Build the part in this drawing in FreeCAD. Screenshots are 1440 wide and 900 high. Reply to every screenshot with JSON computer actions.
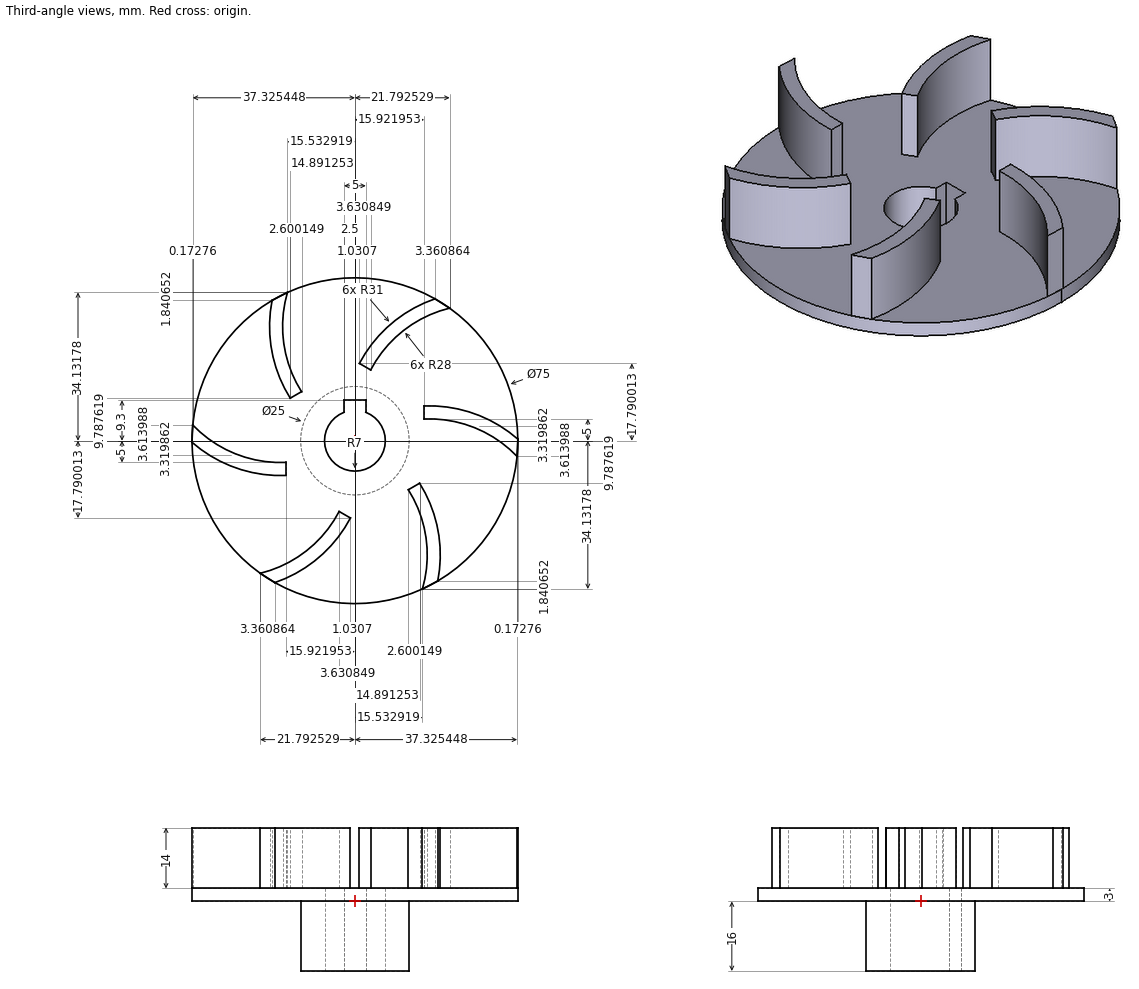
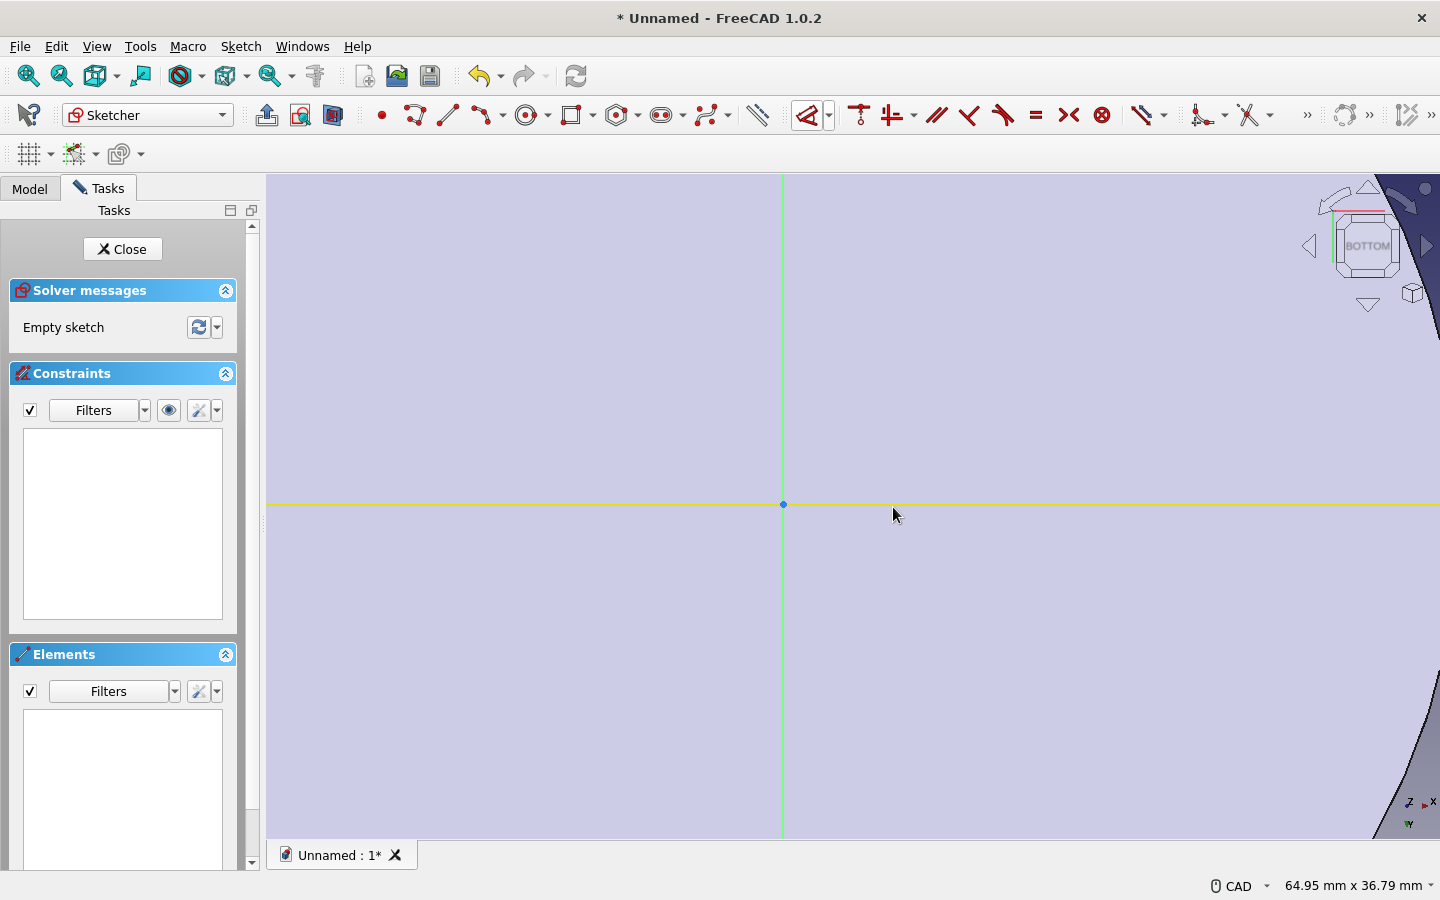
{"action": "key", "text": "g c"}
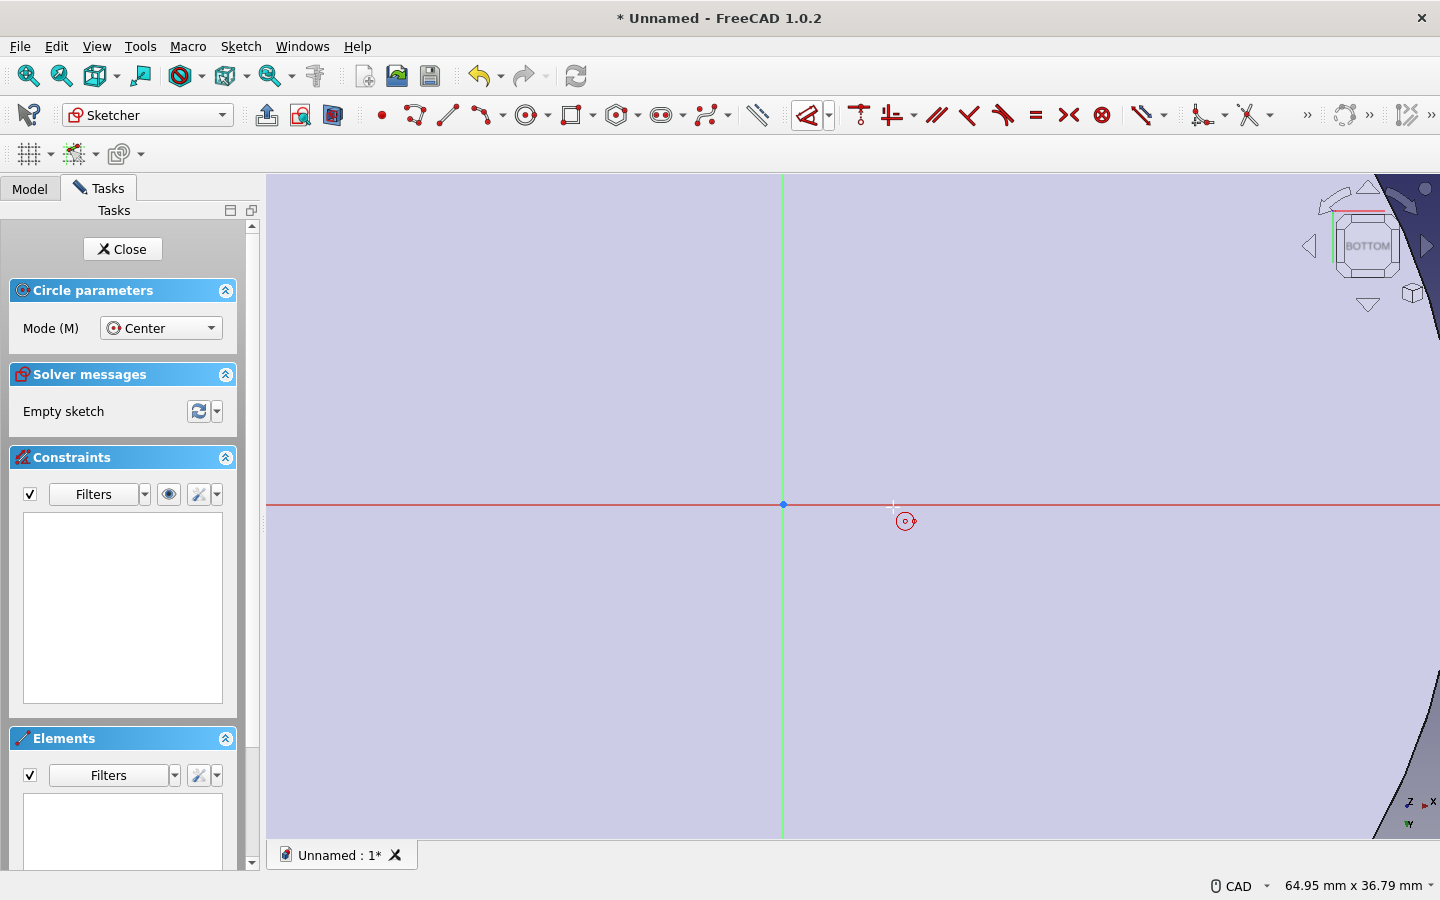
{"action": "left_click", "coordinate": [783, 505]}
{"action": "mouse_move", "coordinate": [943, 345]}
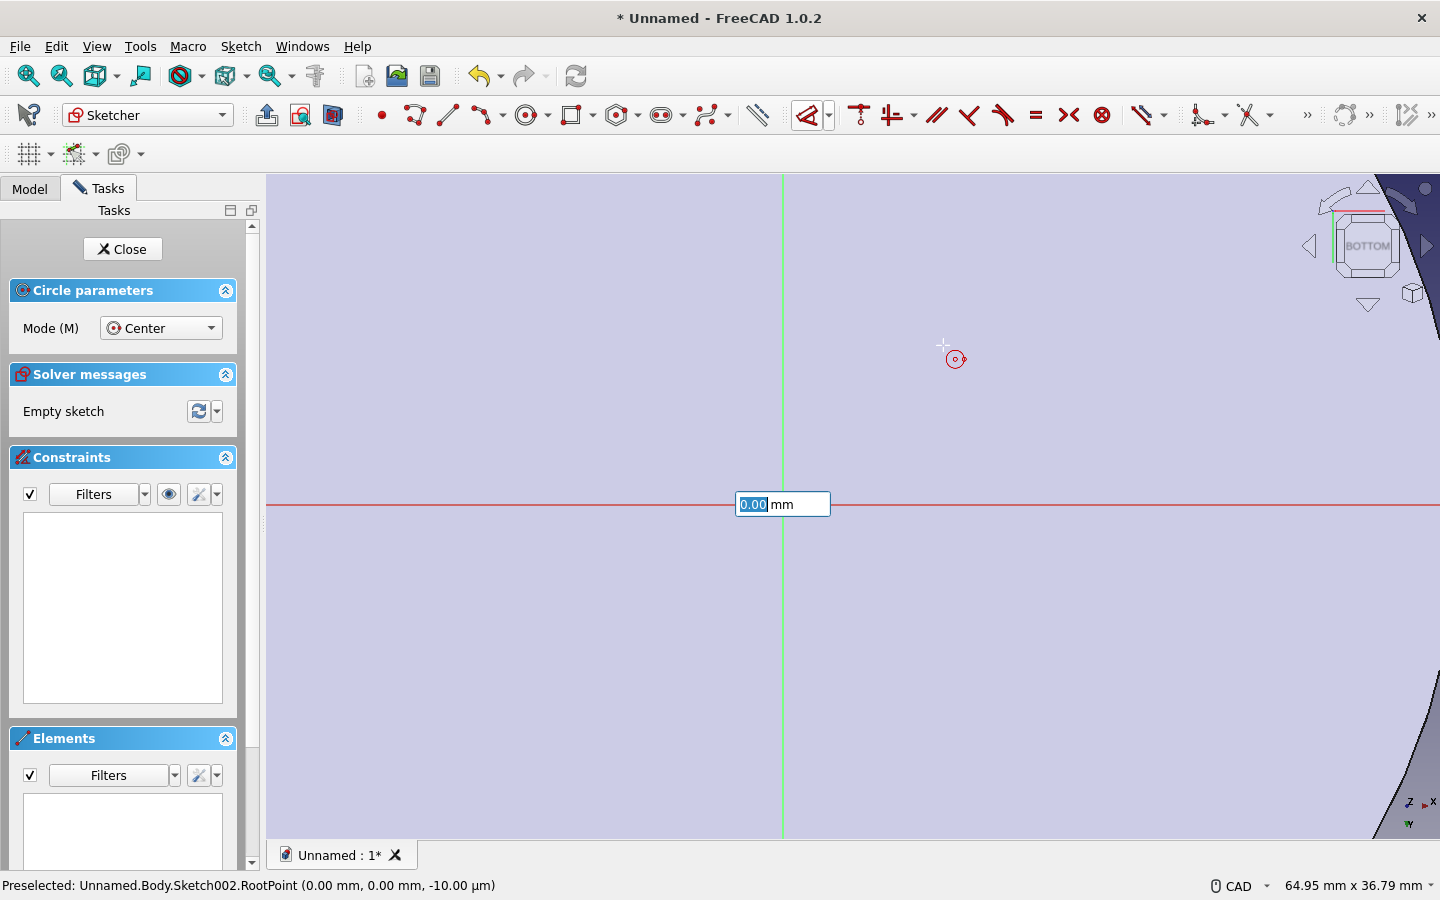
{"action": "type", "text": "25"}
{"action": "key", "text": "Return"}
{"action": "key", "text": "Escape"}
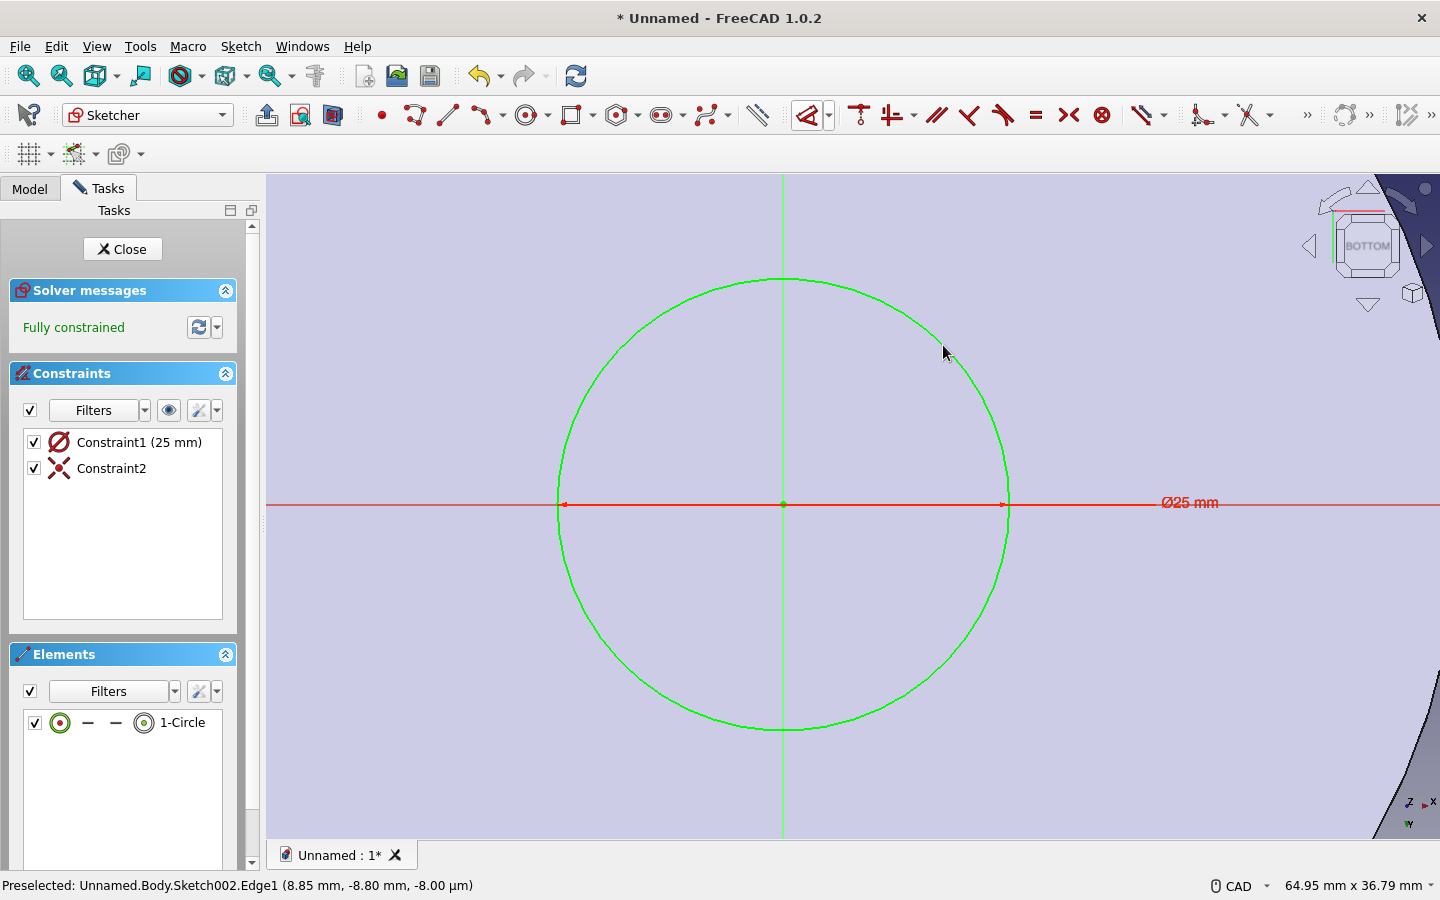
{"action": "left_click", "coordinate": [123, 249]}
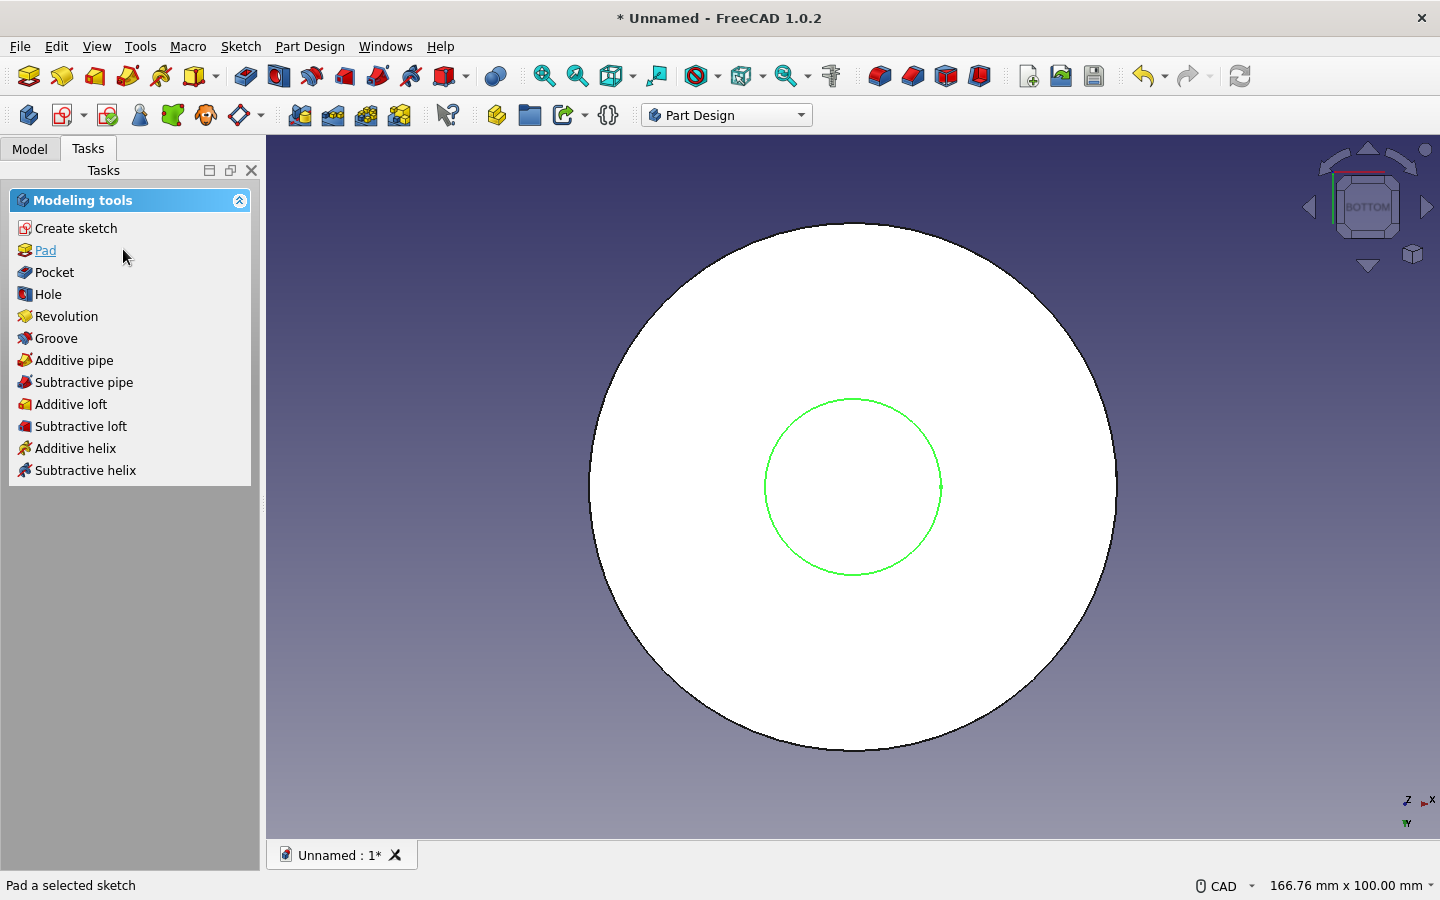
{"action": "left_click", "coordinate": [29, 76]}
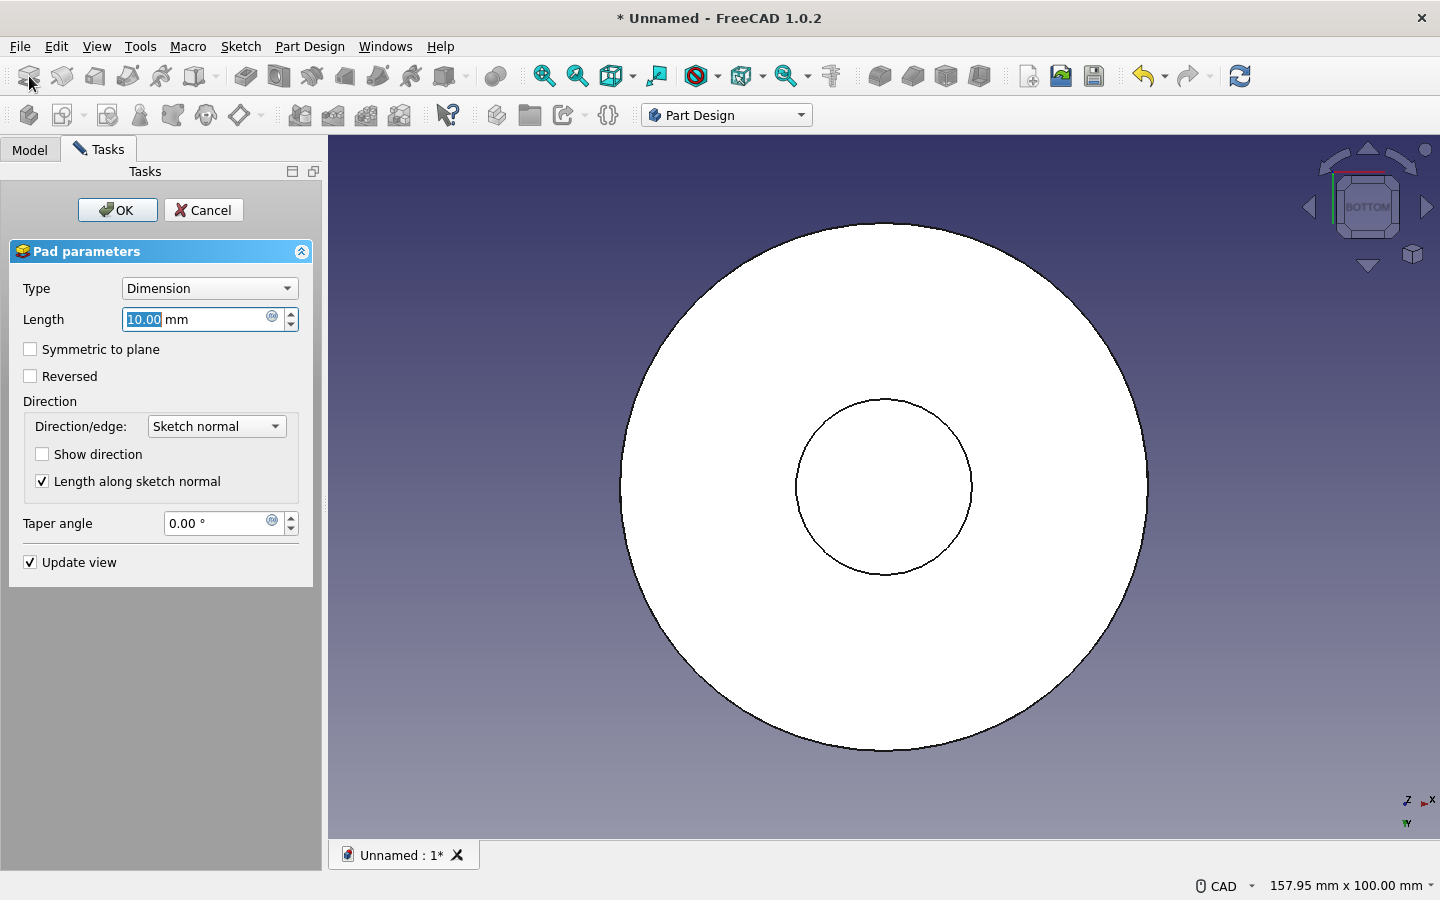
{"action": "type", "text": "16"}
{"action": "key", "text": "Tab"}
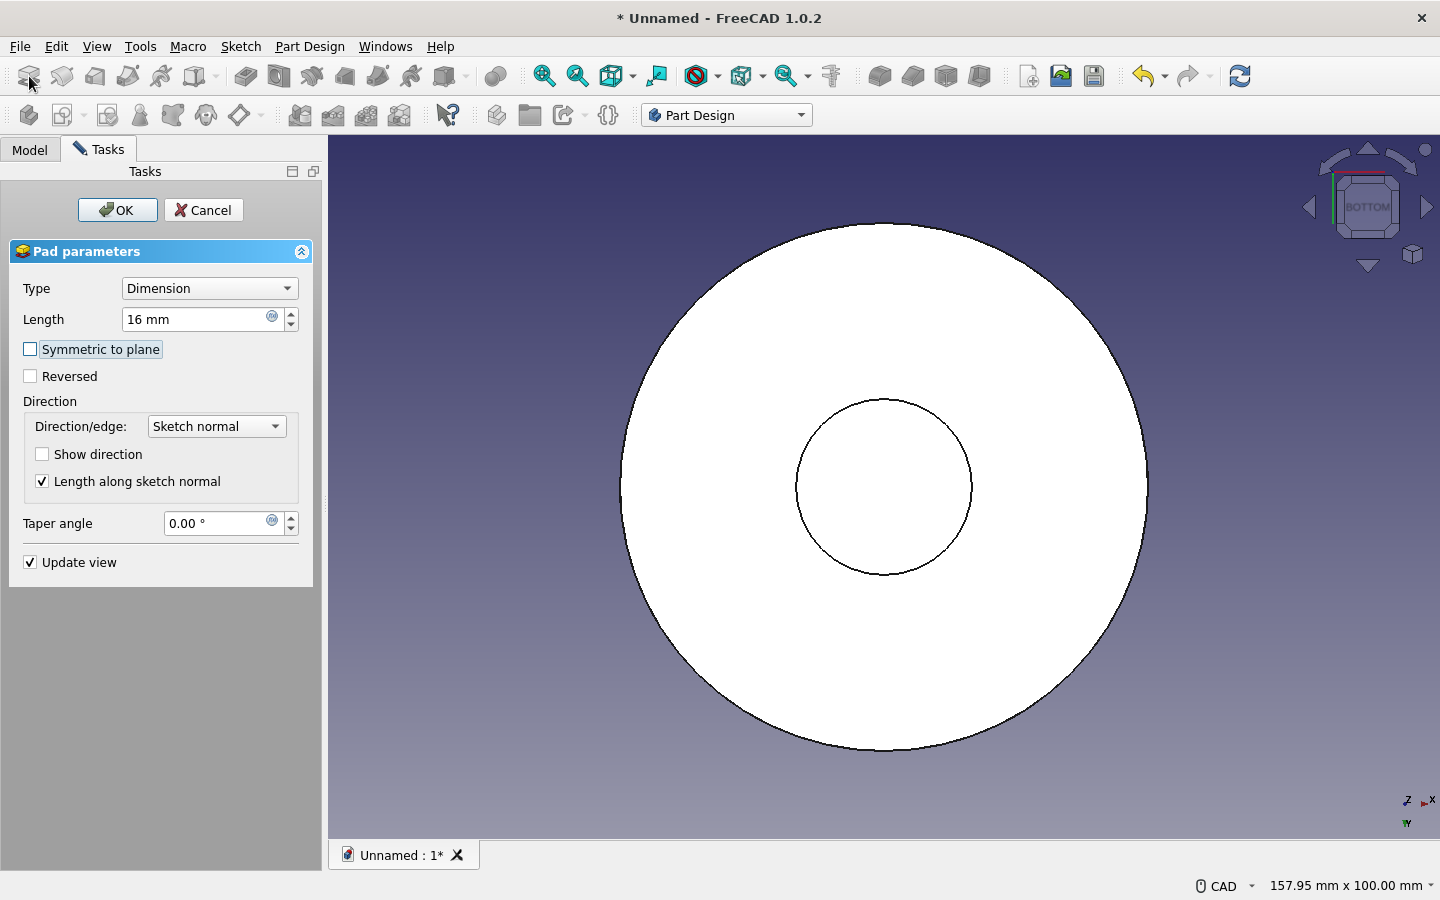
{"action": "left_click", "coordinate": [118, 210]}